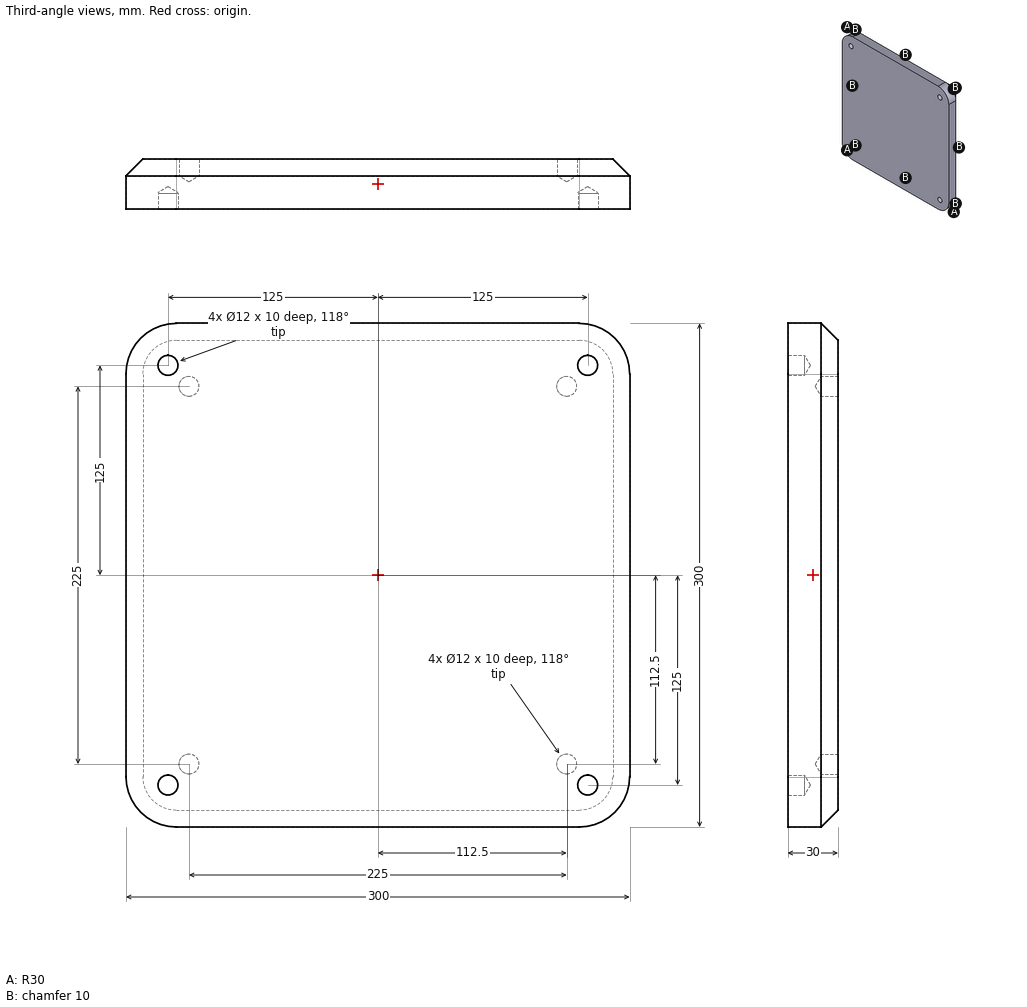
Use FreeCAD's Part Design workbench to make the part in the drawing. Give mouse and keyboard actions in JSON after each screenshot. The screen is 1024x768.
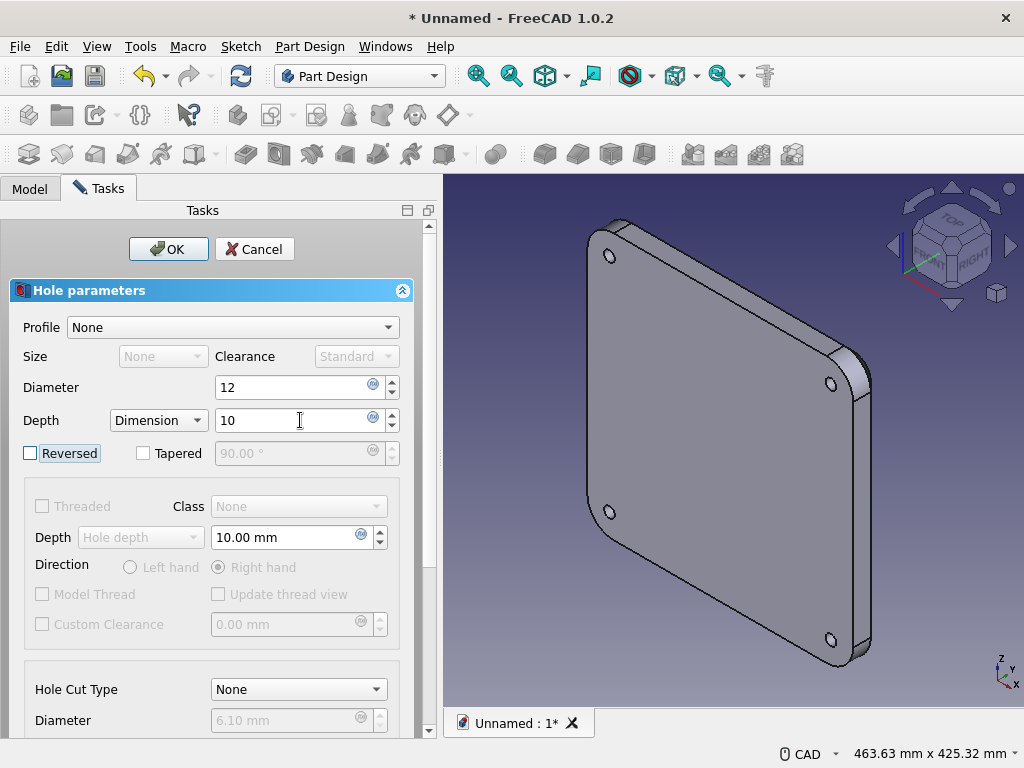
{"action": "left_click", "coordinate": [169, 249]}